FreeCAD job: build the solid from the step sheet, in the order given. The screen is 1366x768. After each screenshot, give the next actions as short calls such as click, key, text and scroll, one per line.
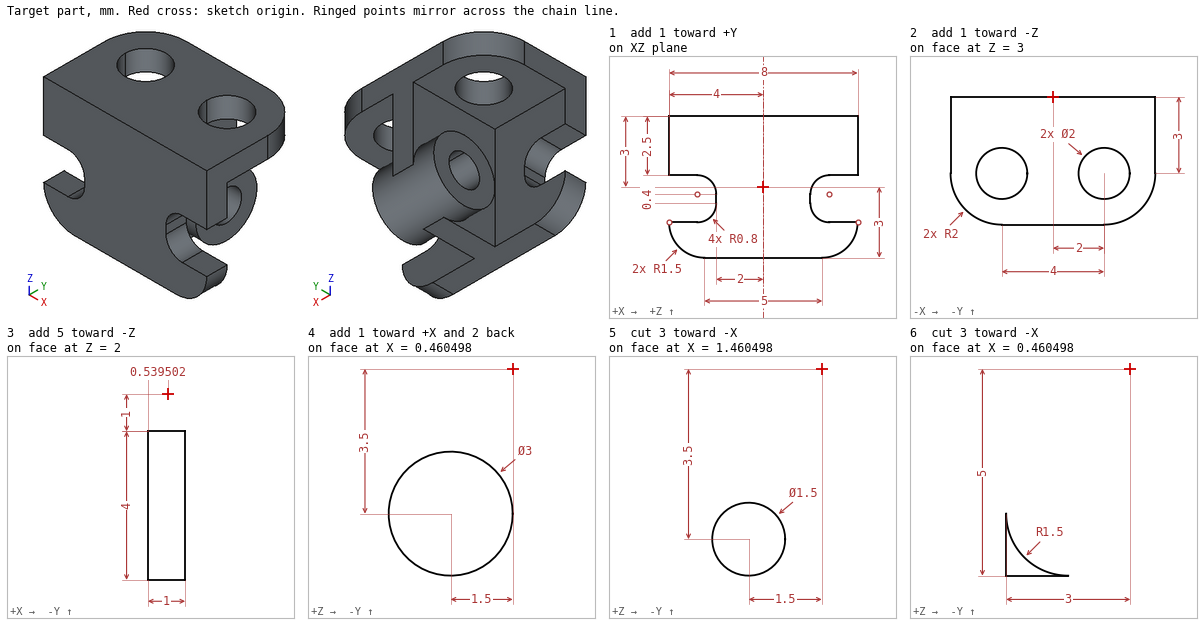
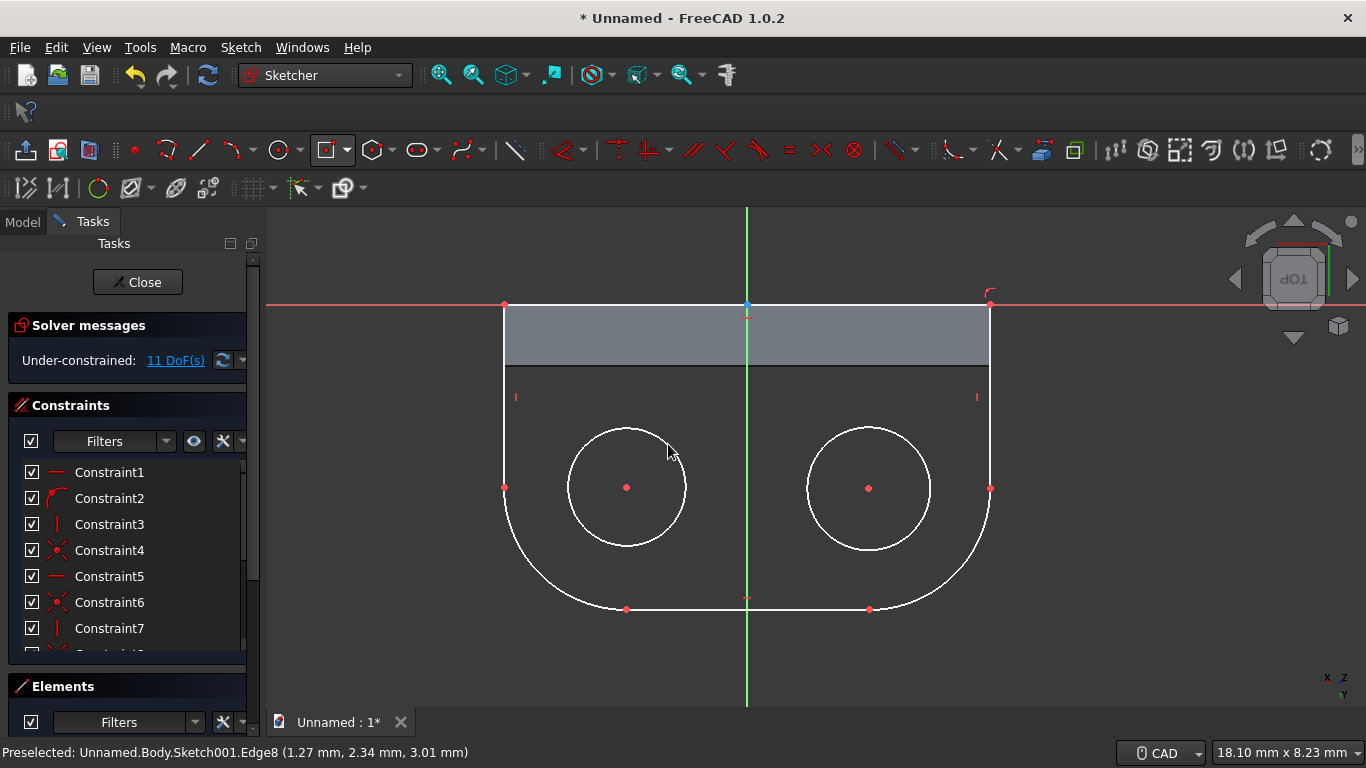
click(699, 610)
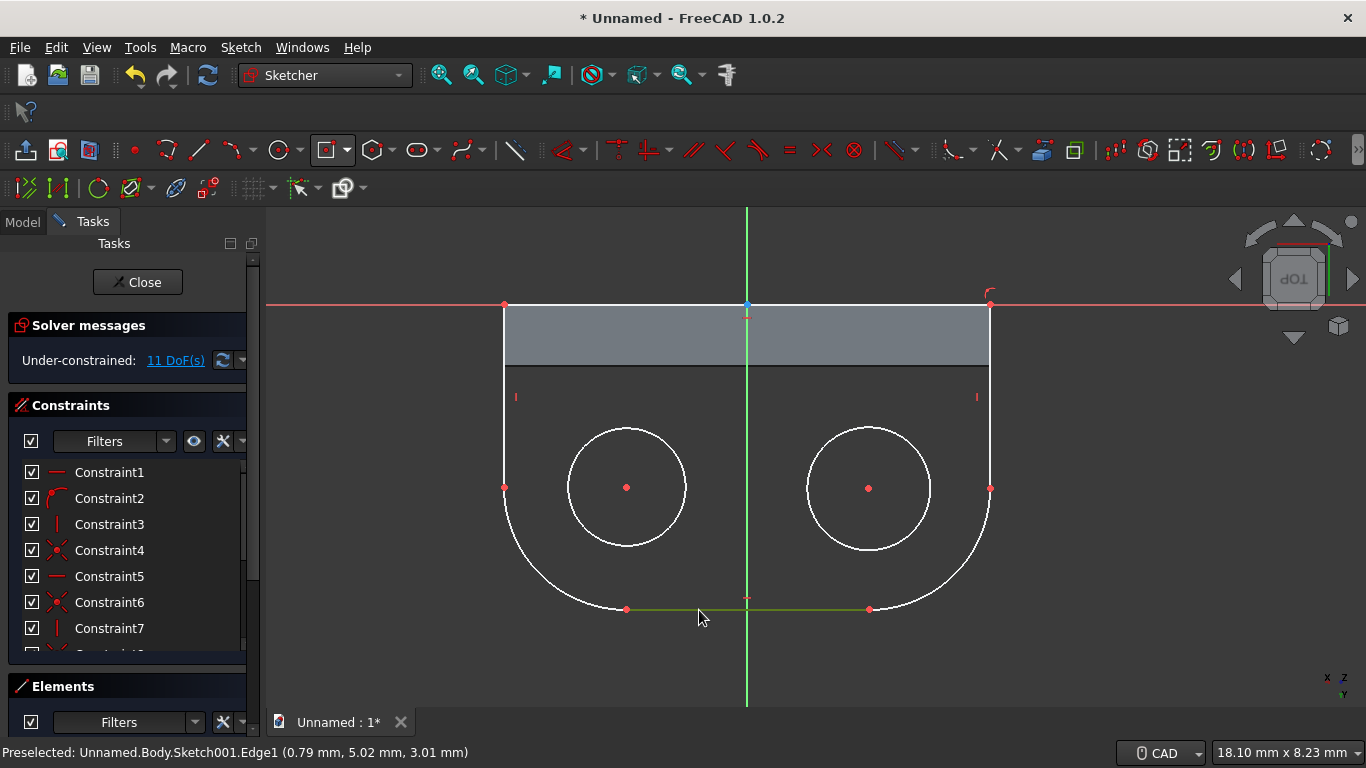
click(924, 597)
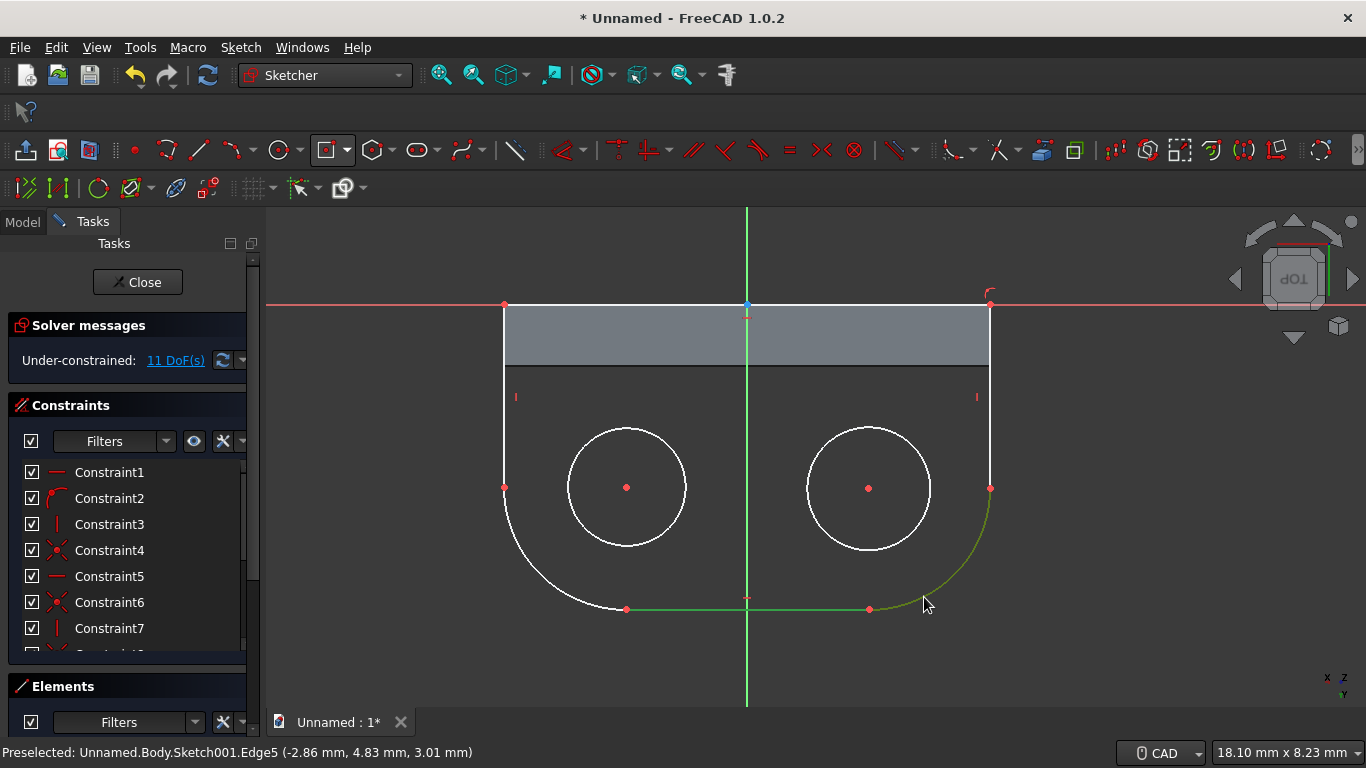
click(758, 150)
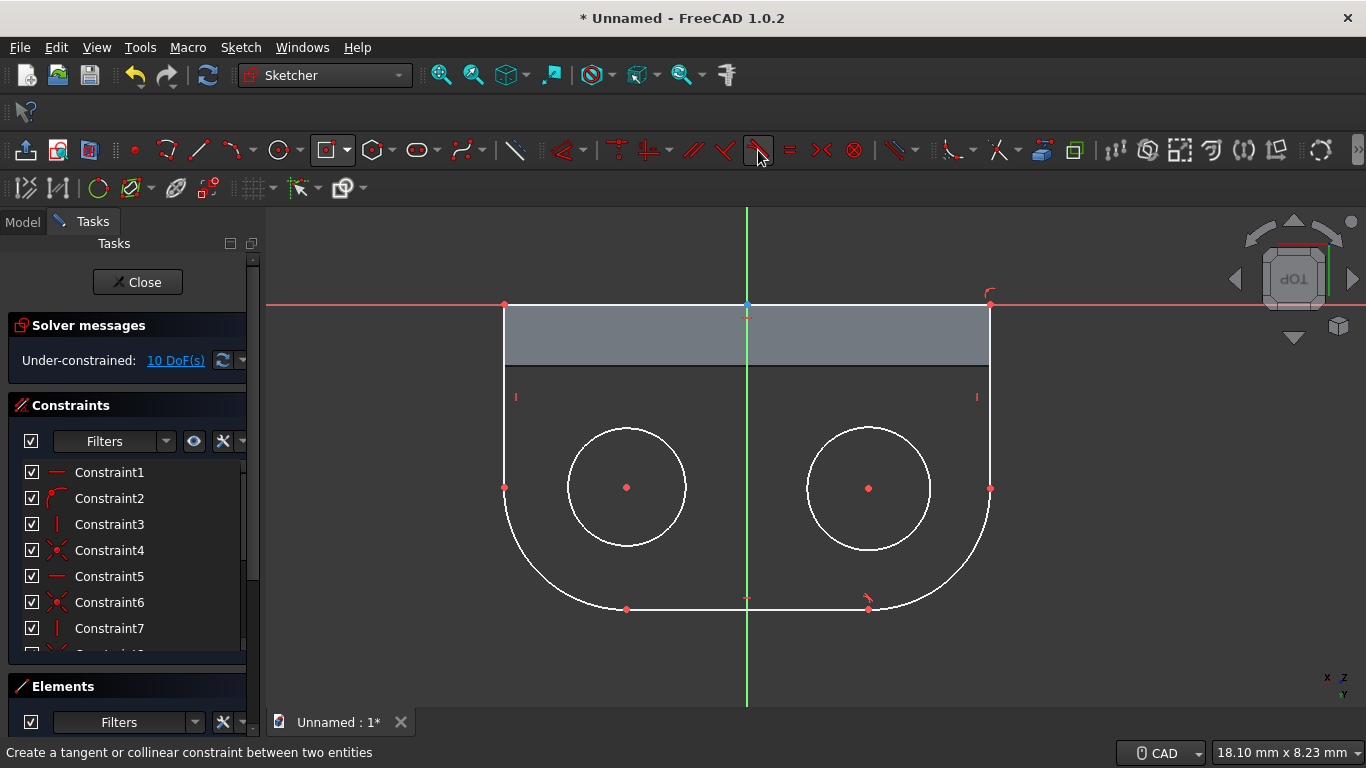
click(699, 610)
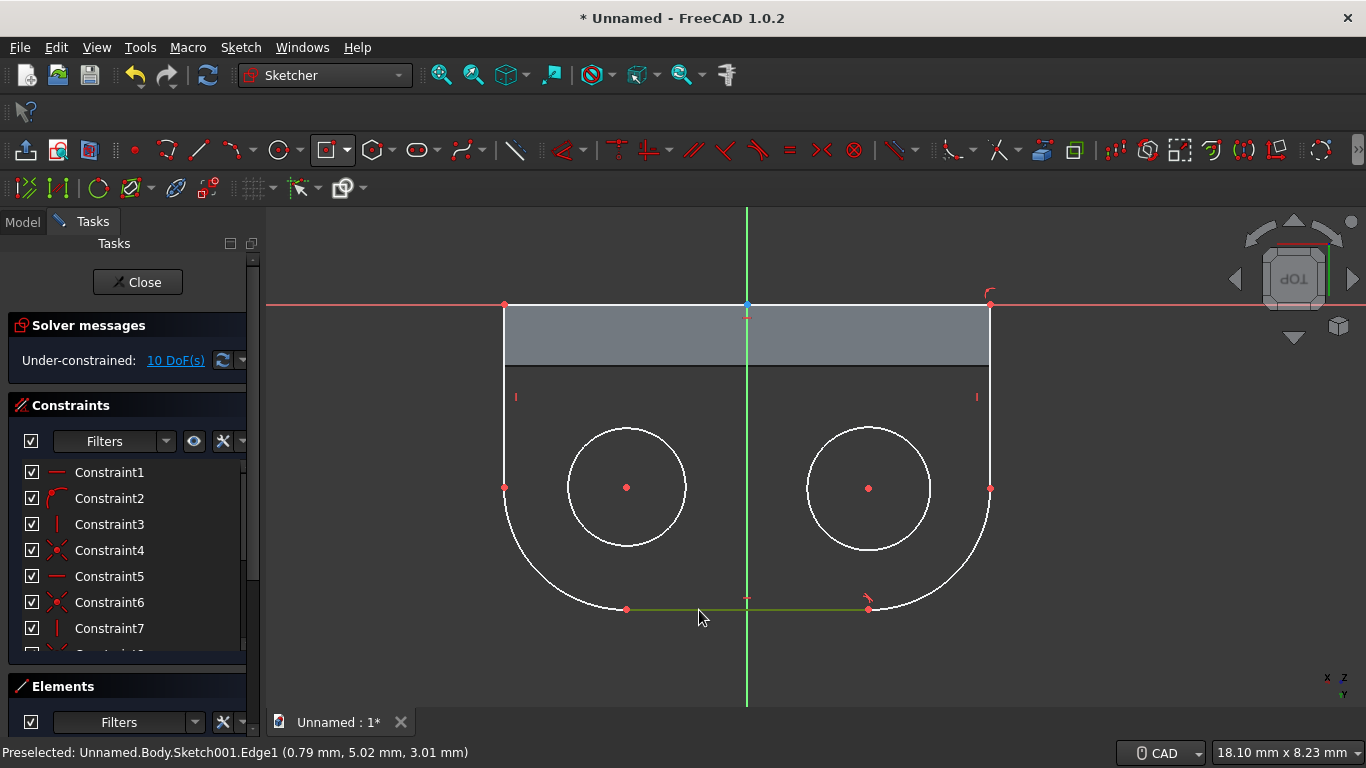
click(518, 543)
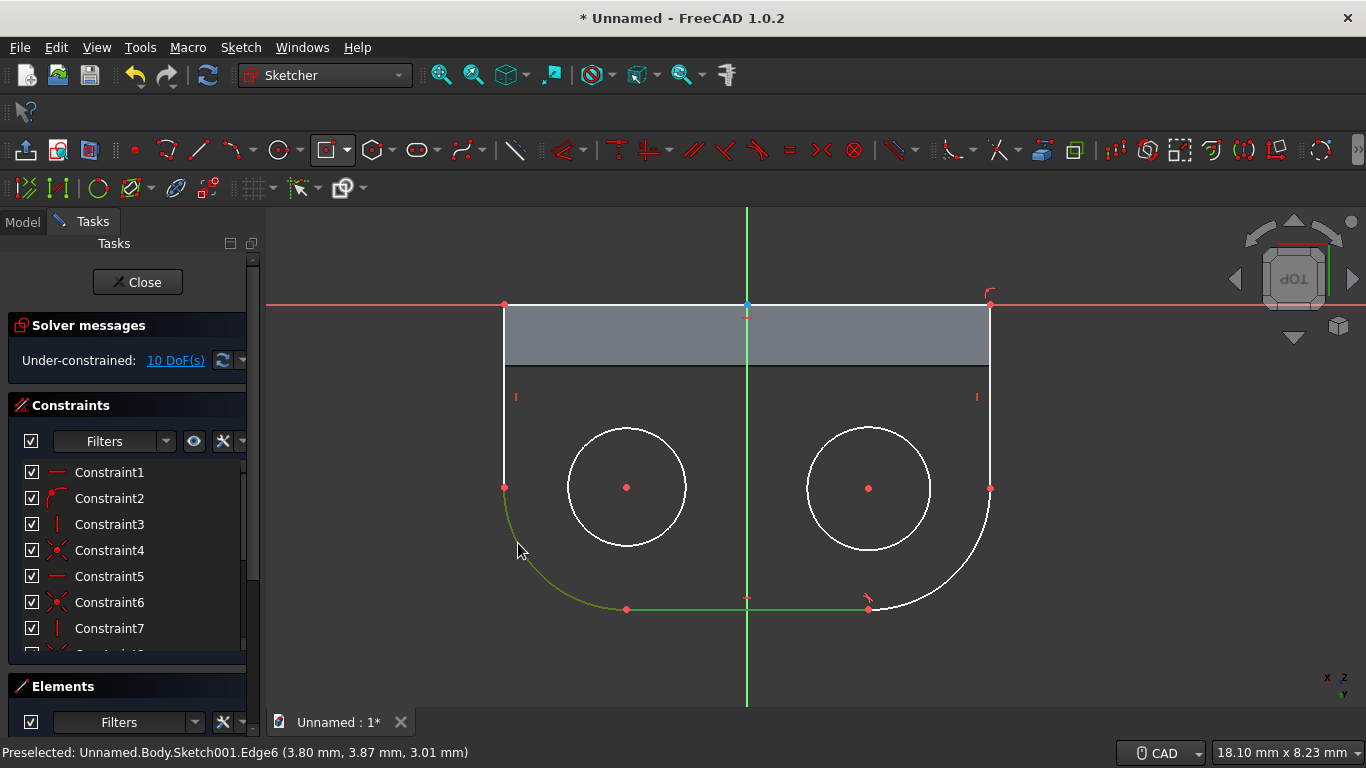
click(758, 150)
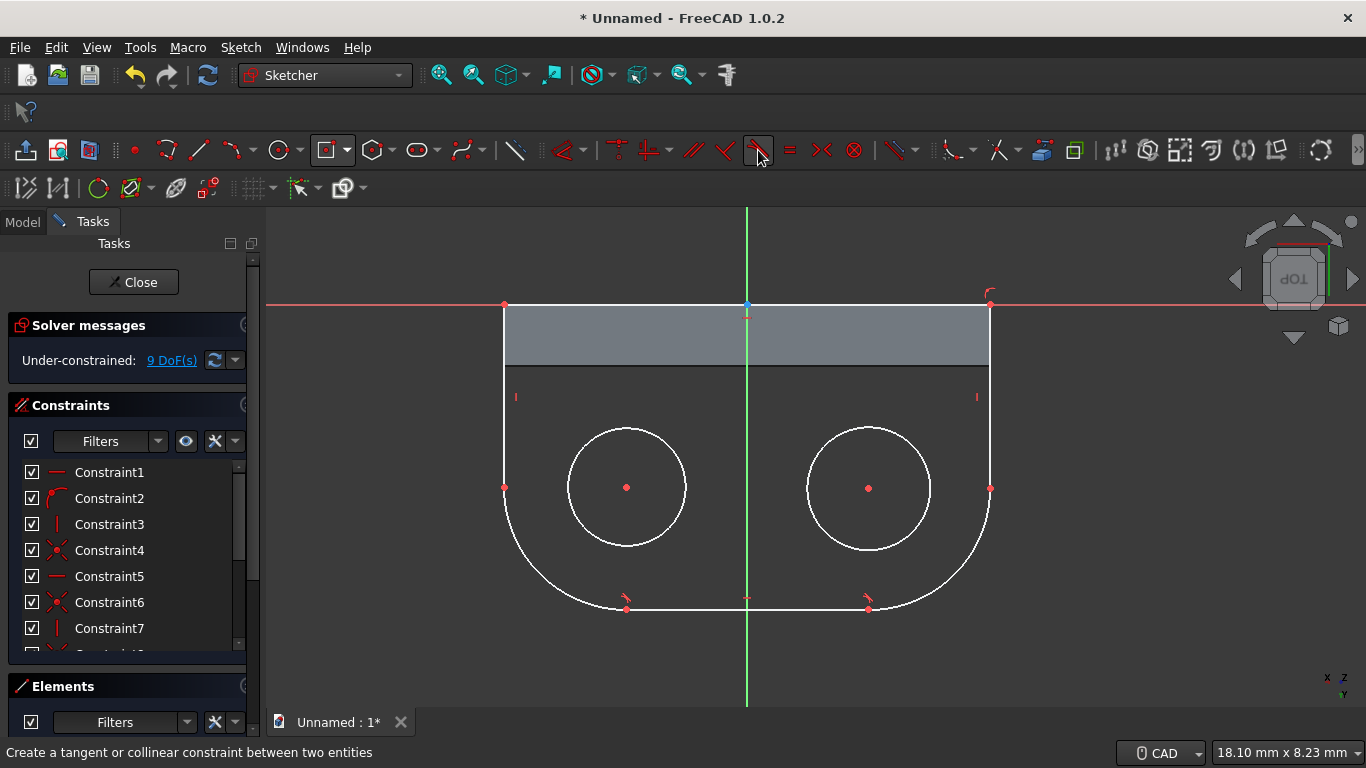
click(990, 433)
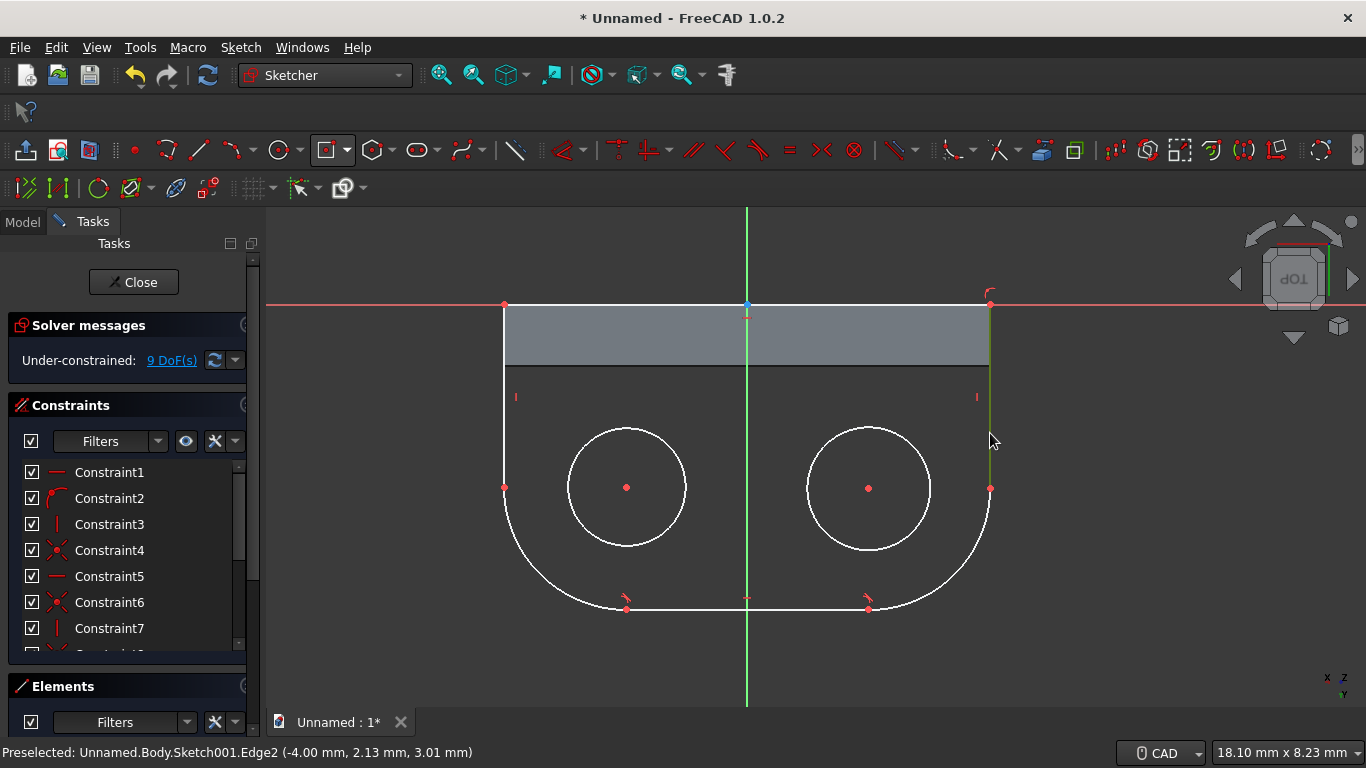
click(924, 597)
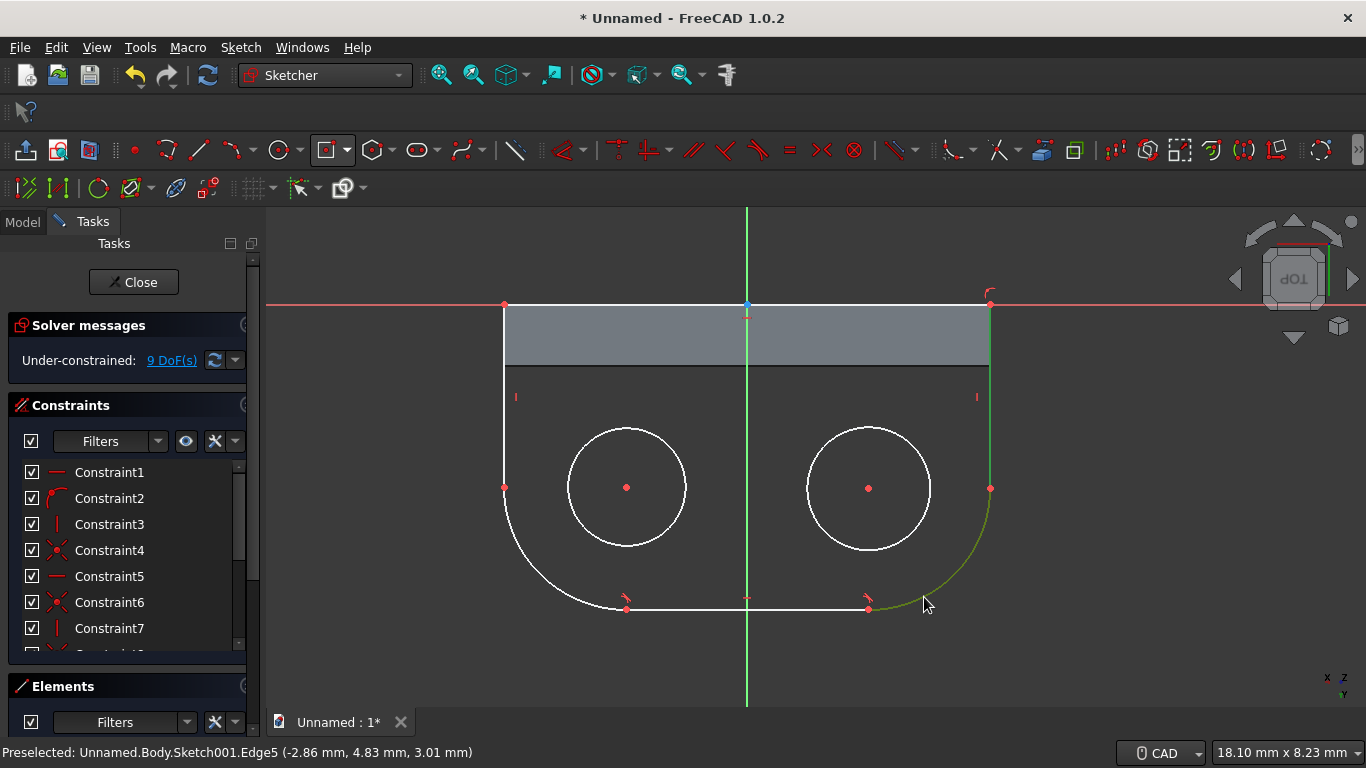
click(758, 150)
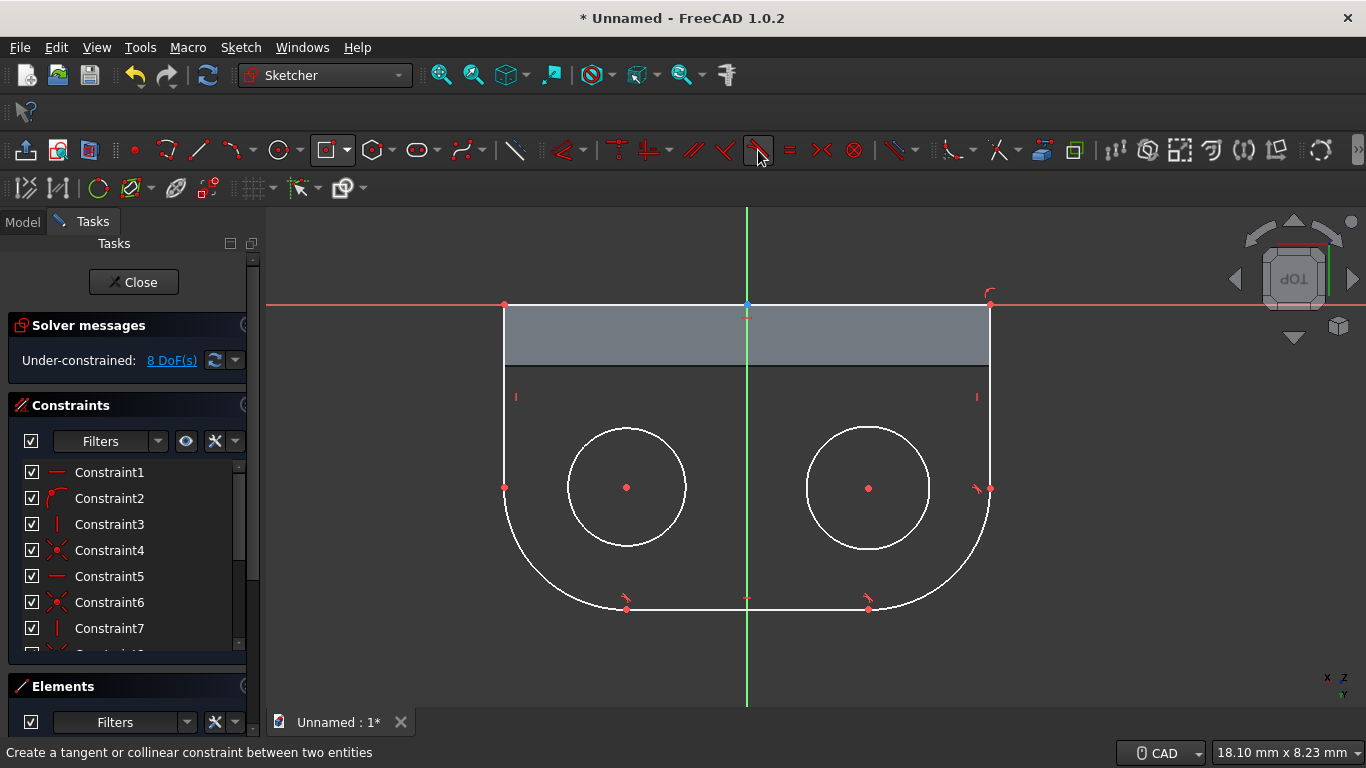
click(504, 360)